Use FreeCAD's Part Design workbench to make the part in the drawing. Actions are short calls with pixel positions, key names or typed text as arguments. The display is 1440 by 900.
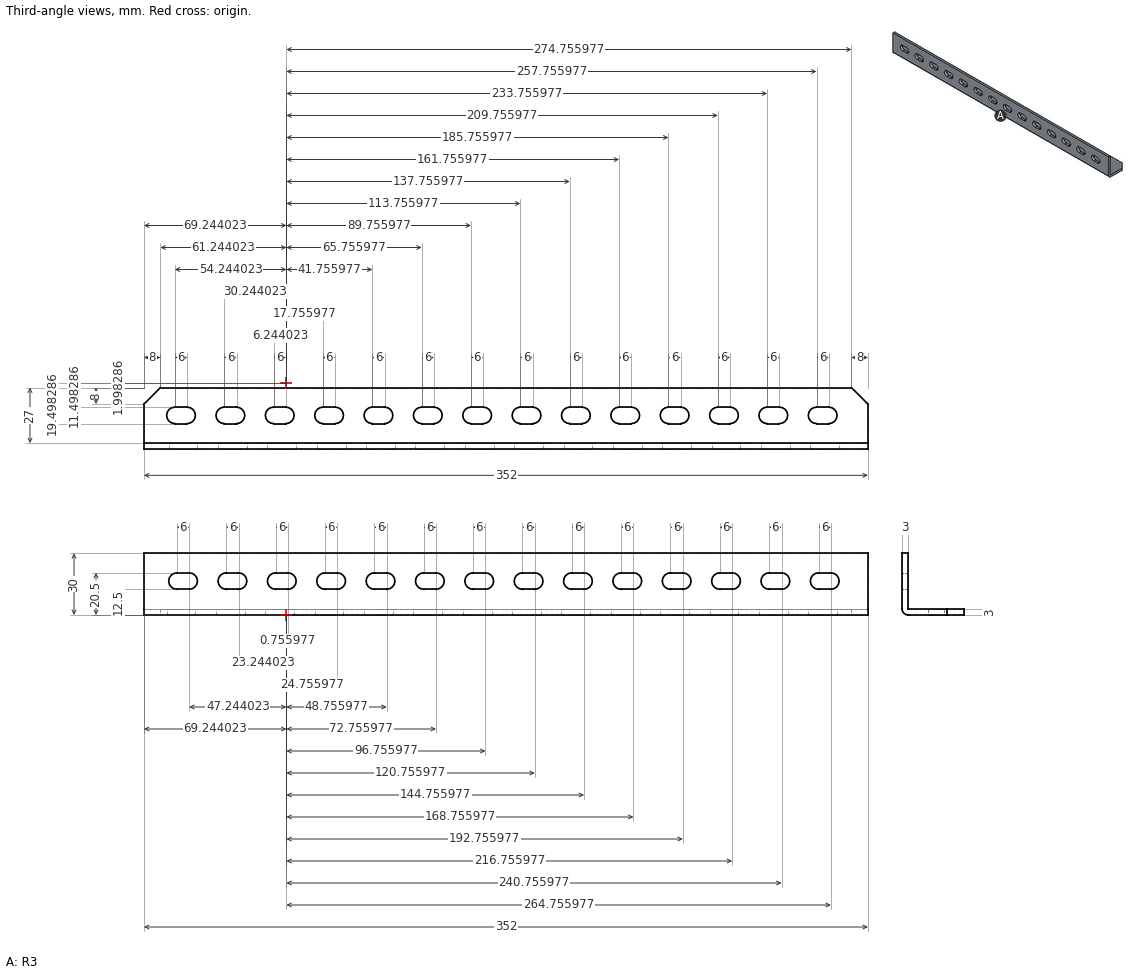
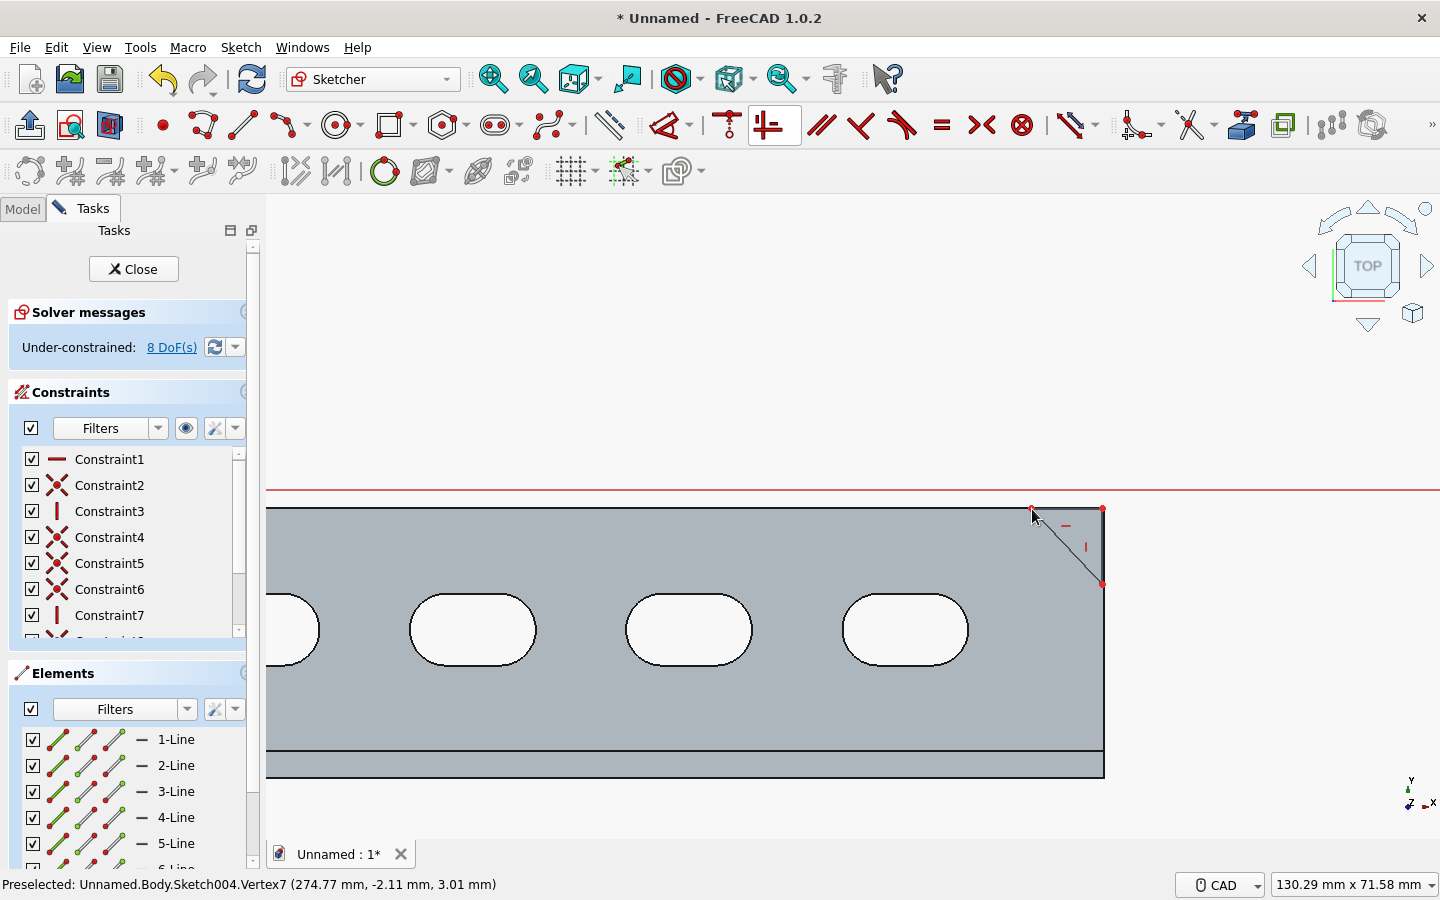
click(664, 126)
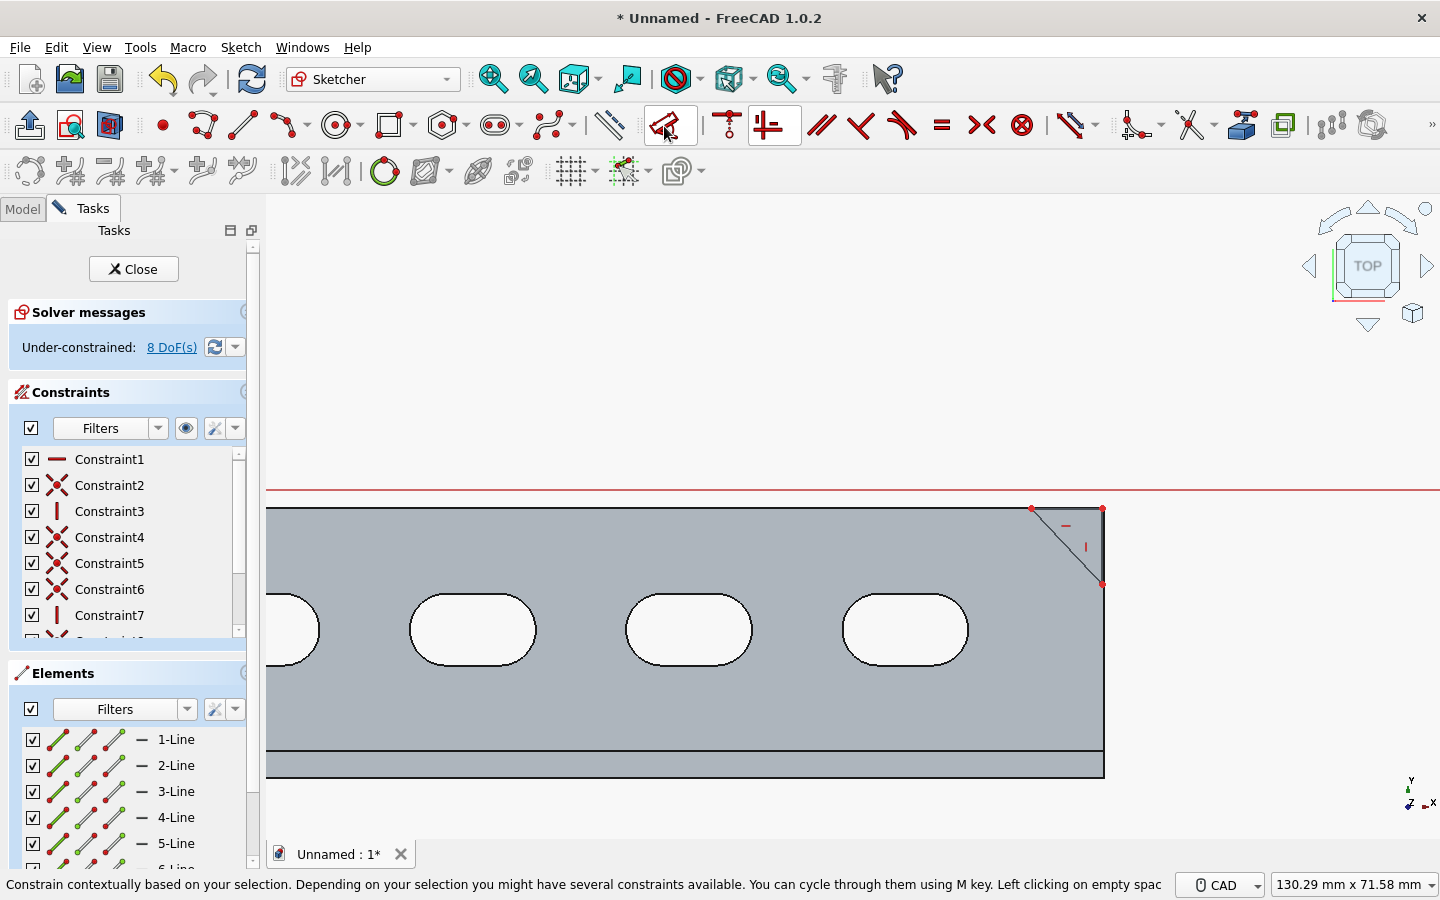
scroll(1105, 512, down, 8)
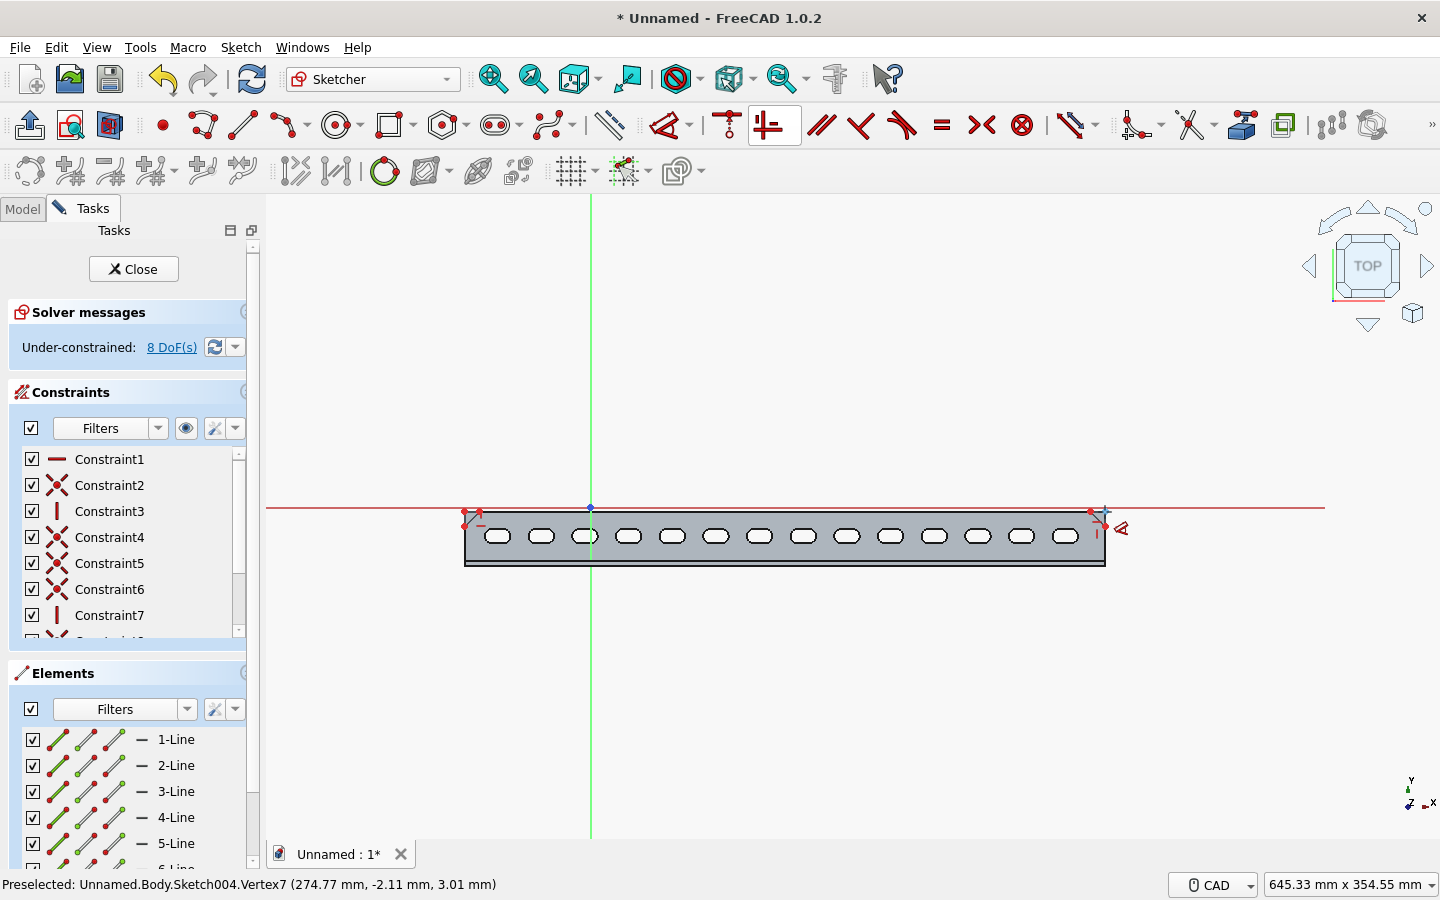
scroll(475, 512, up, 8)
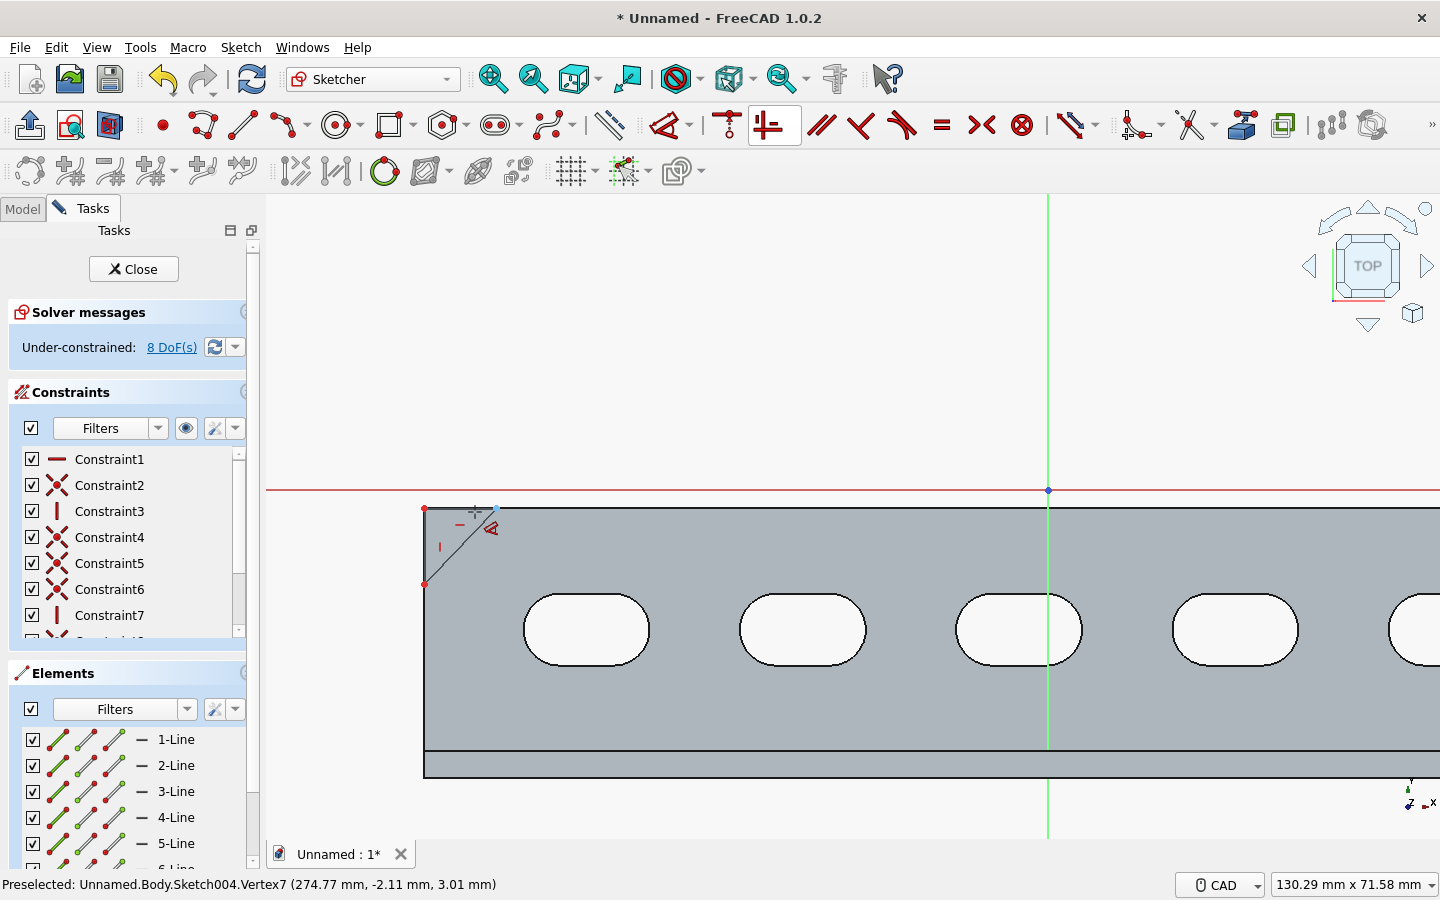
click(475, 509)
click(461, 475)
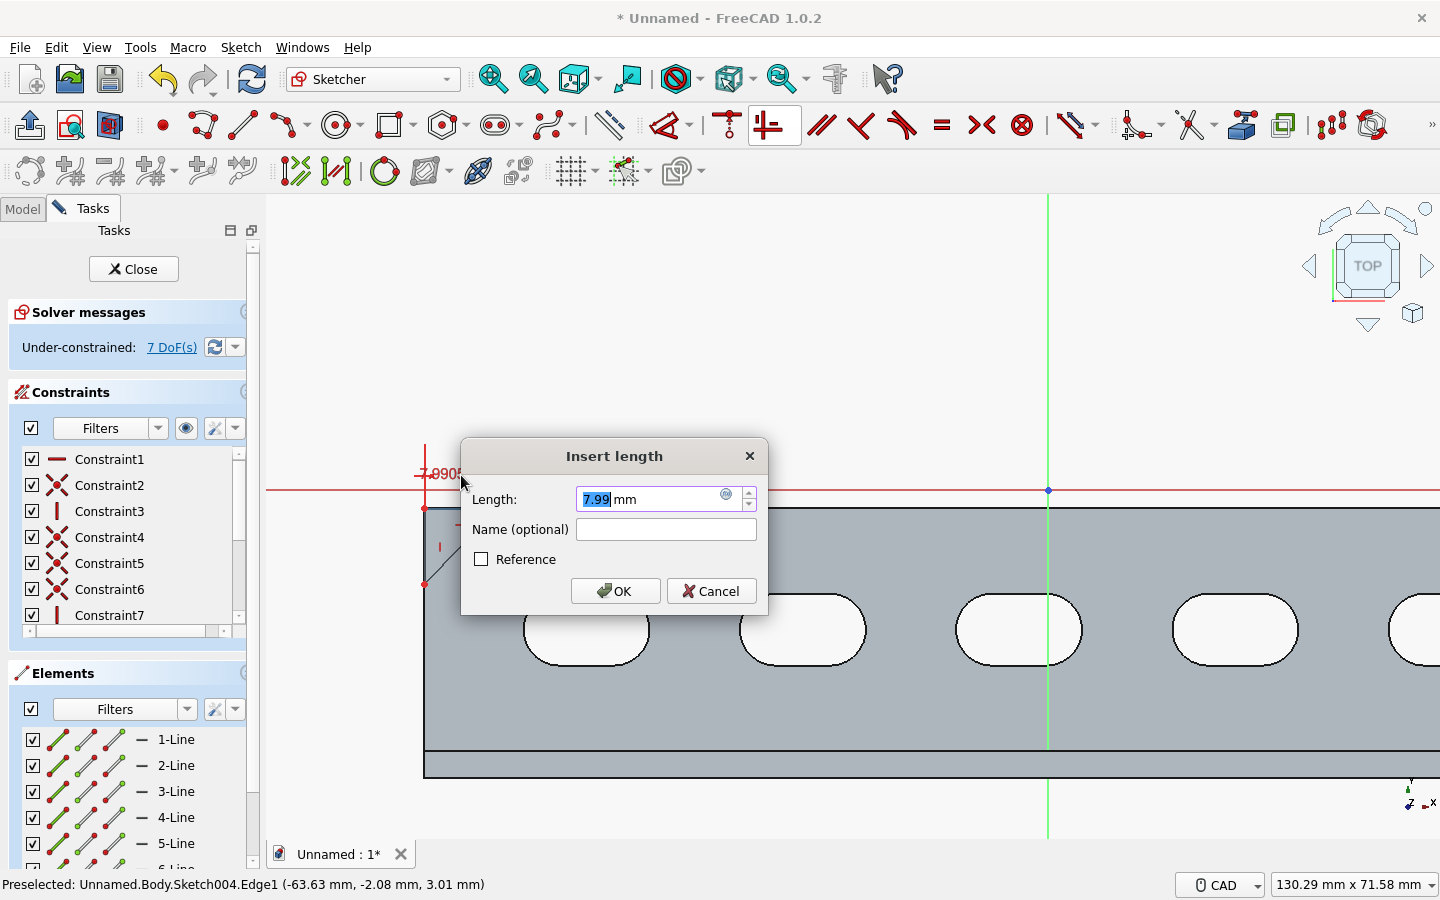
text(8)
key(Return)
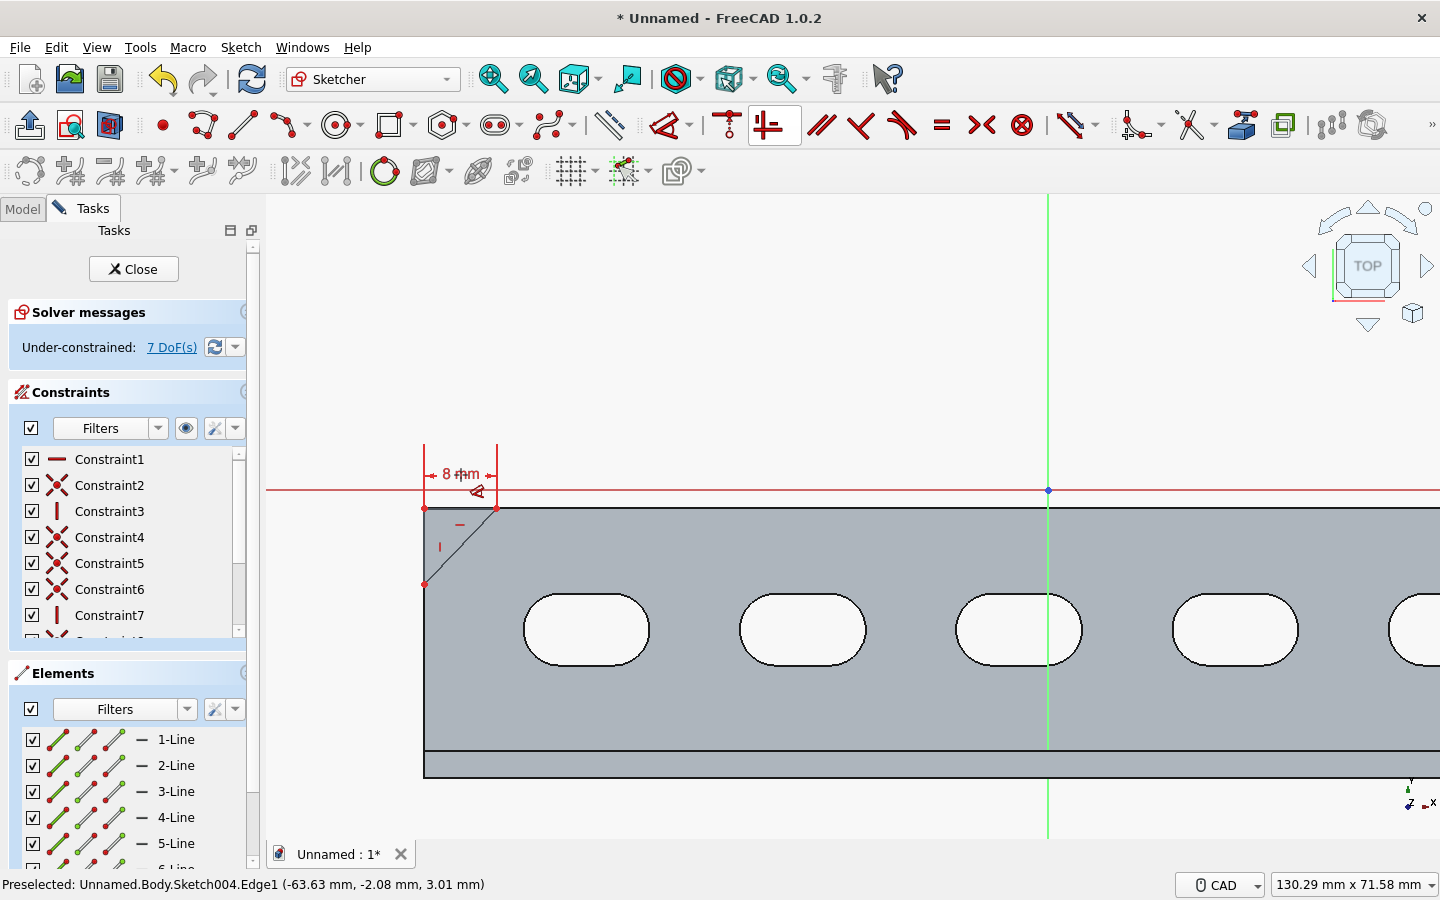
click(424, 531)
click(390, 547)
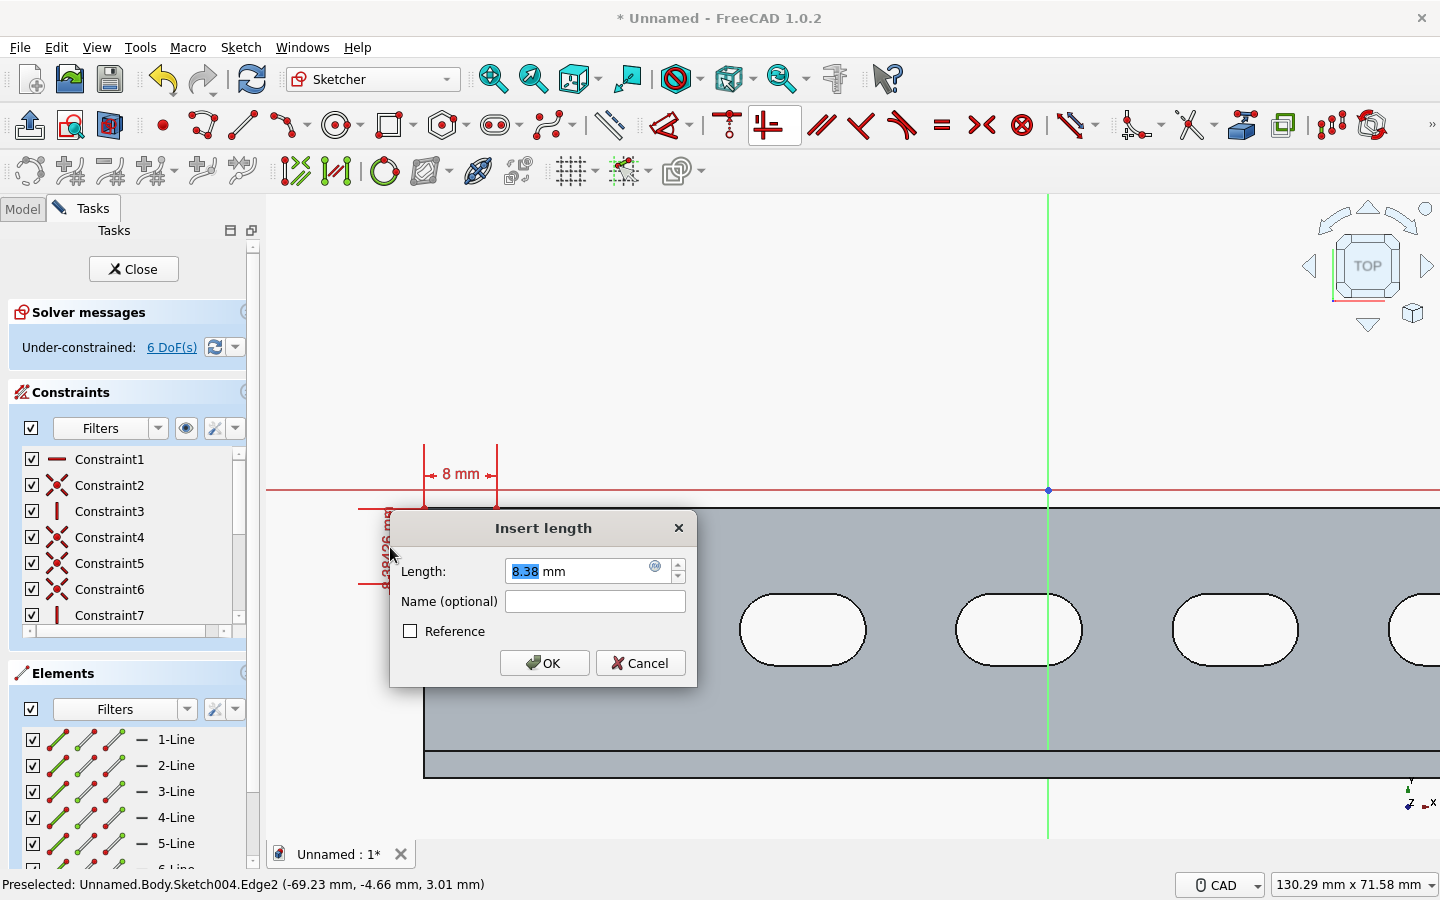
text(8)
key(Return)